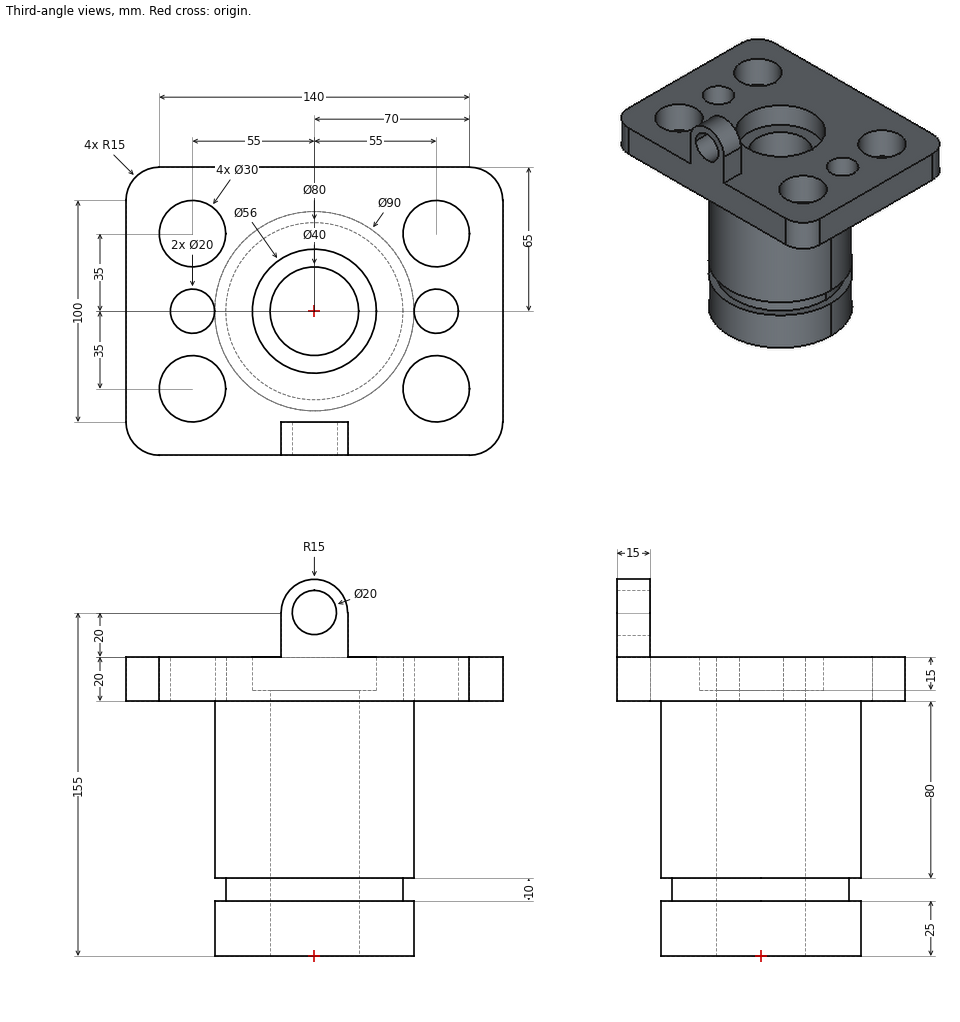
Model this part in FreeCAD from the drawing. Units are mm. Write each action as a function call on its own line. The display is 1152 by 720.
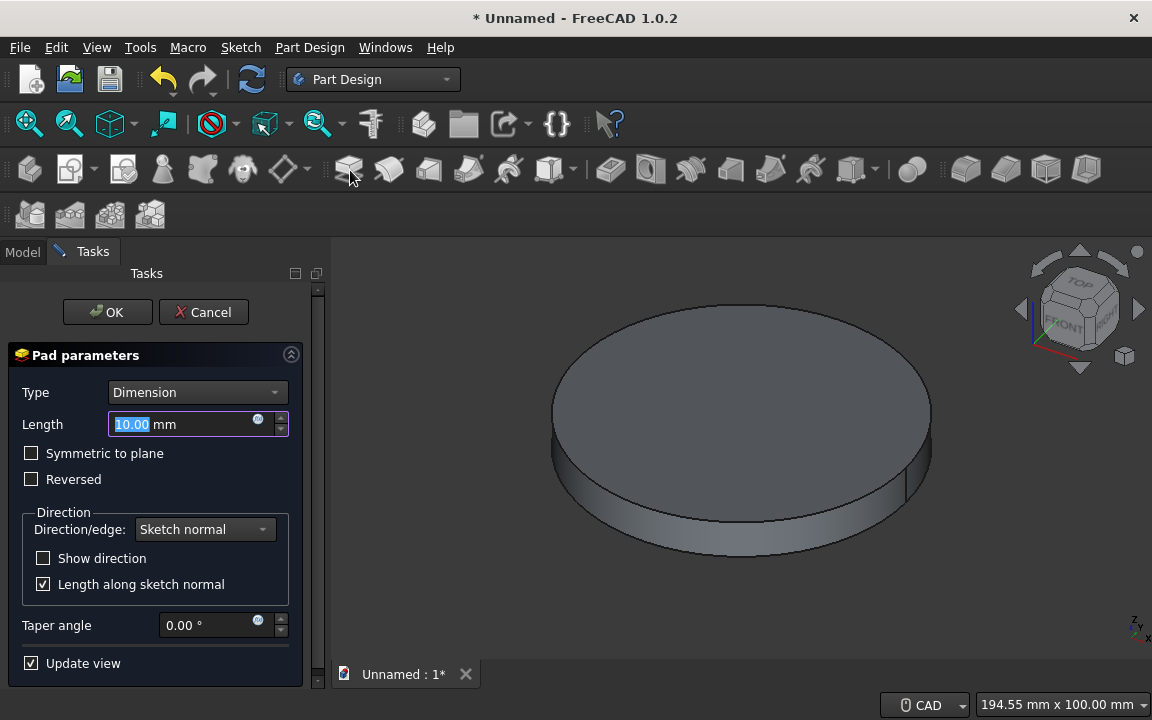
text(25)
key(Tab)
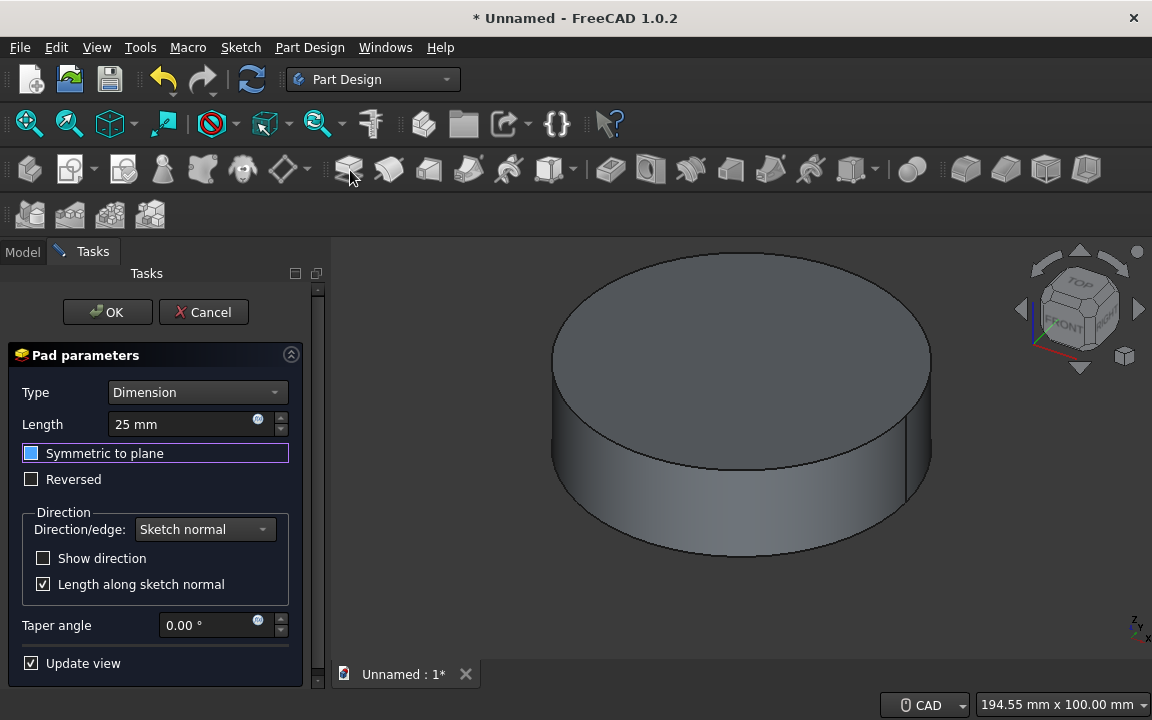
click(108, 312)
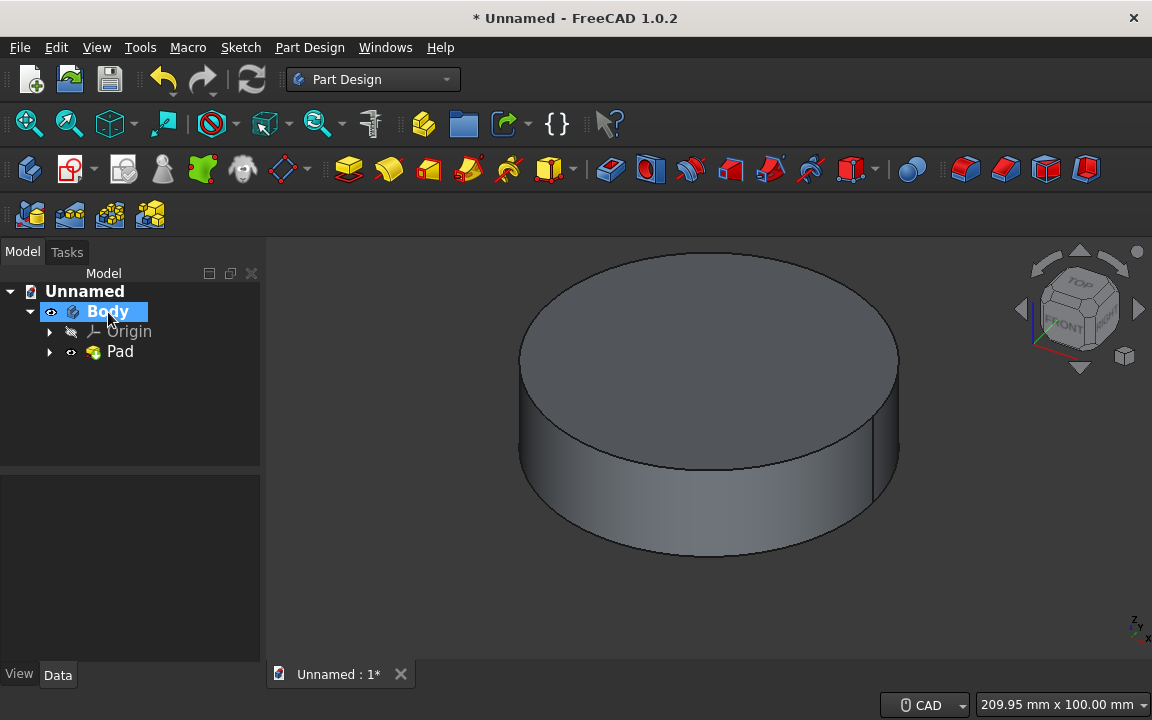
click(30, 124)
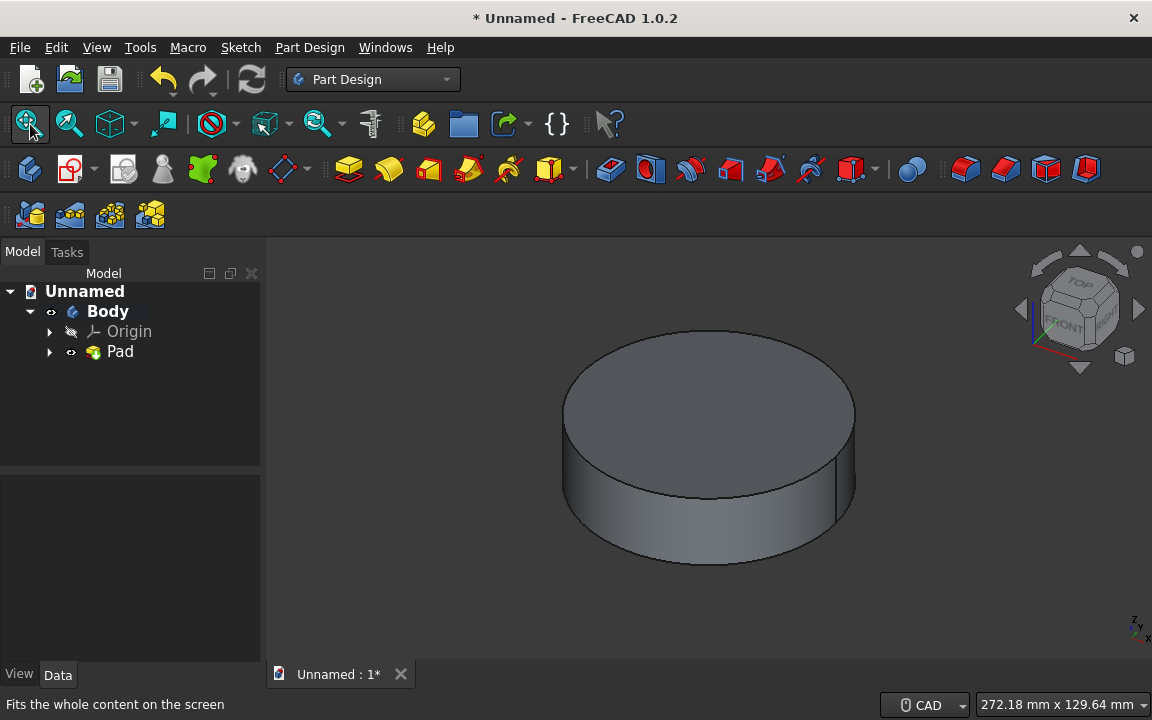
click(709, 414)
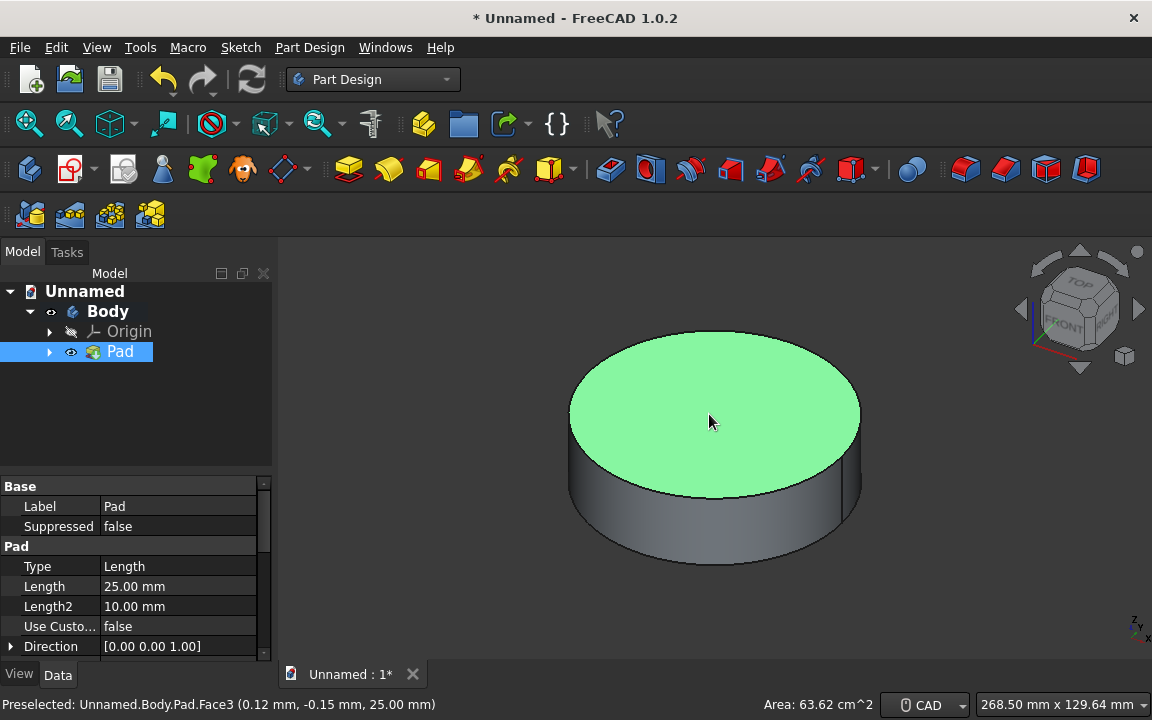
click(70, 170)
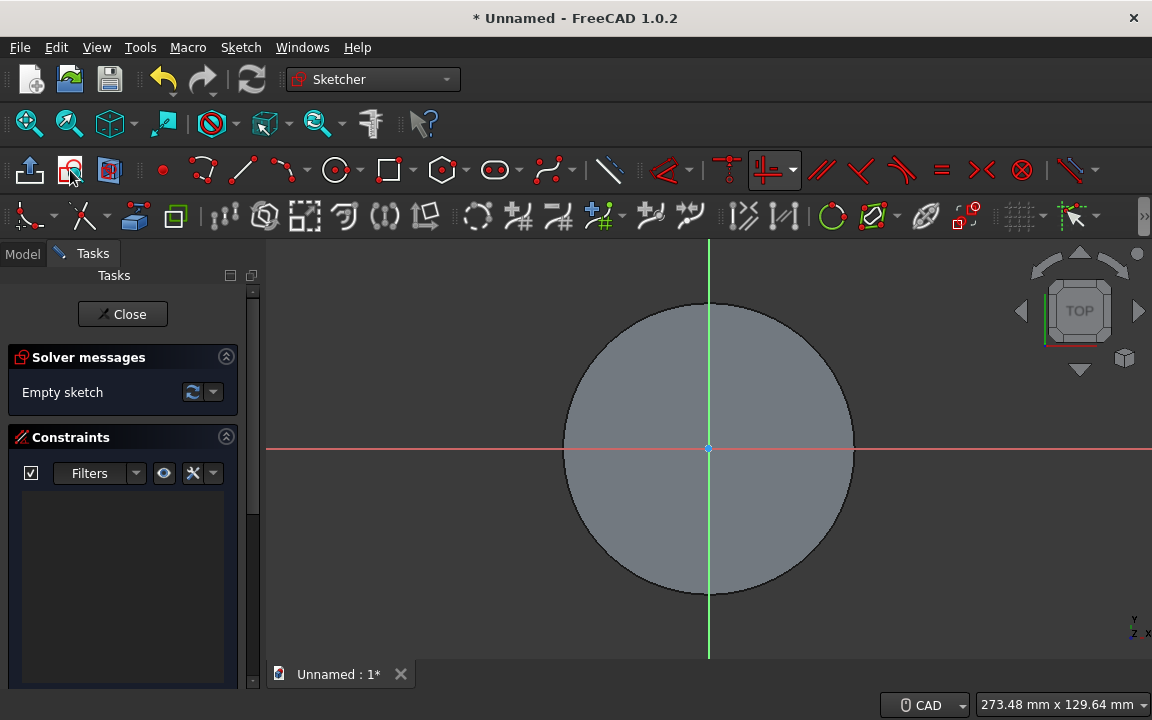
click(336, 170)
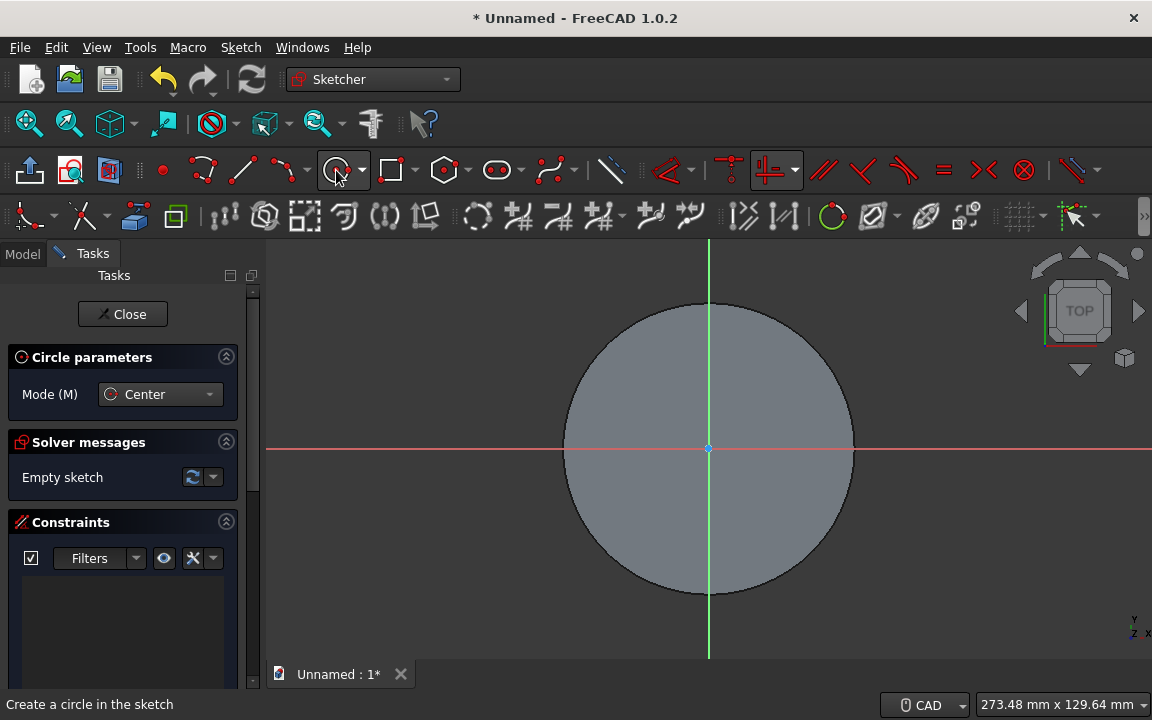
click(709, 449)
click(801, 357)
key(Escape)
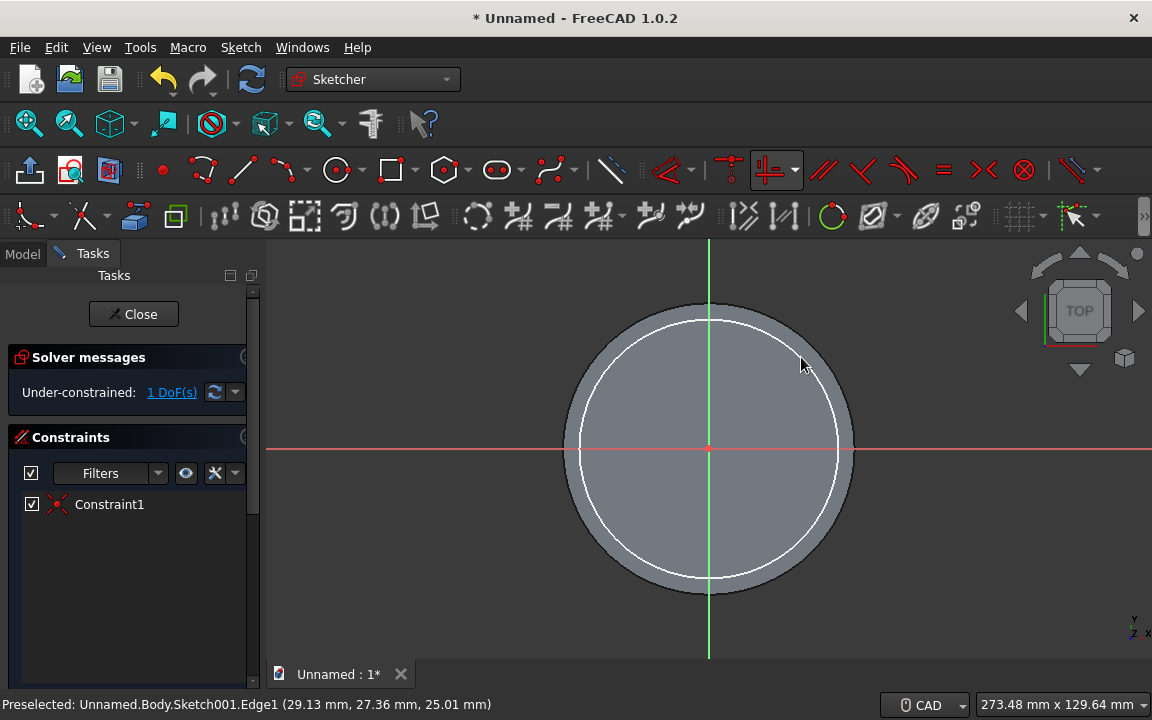
click(666, 170)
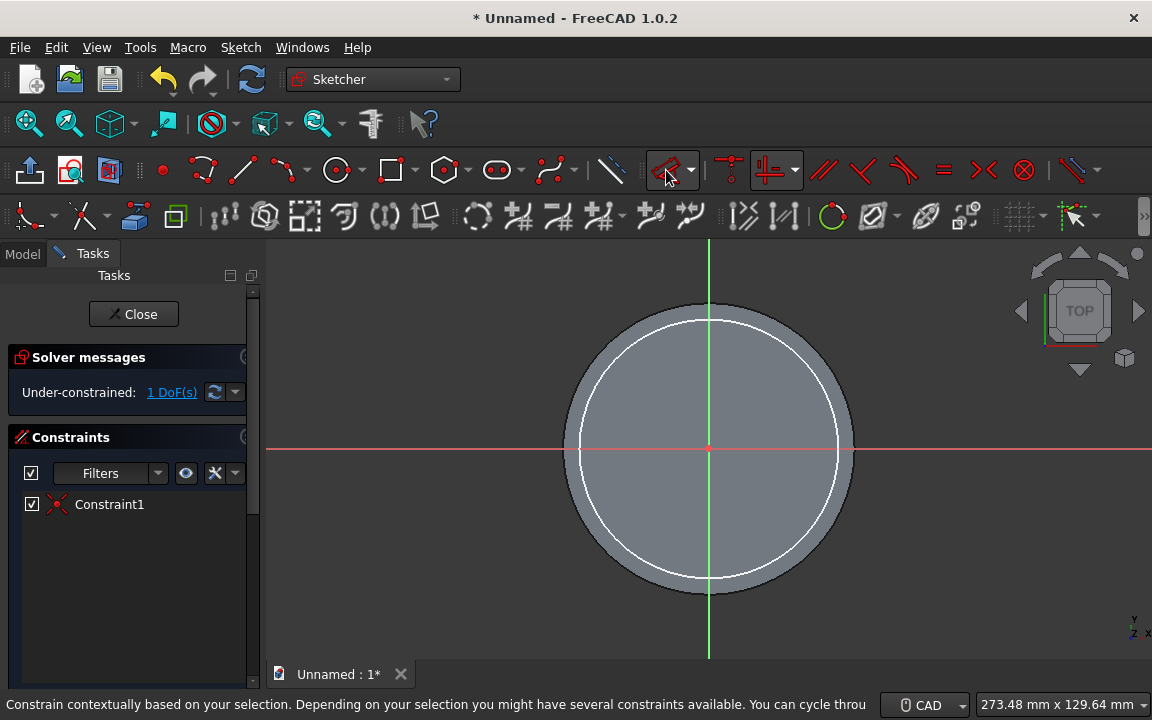
click(800, 357)
click(823, 334)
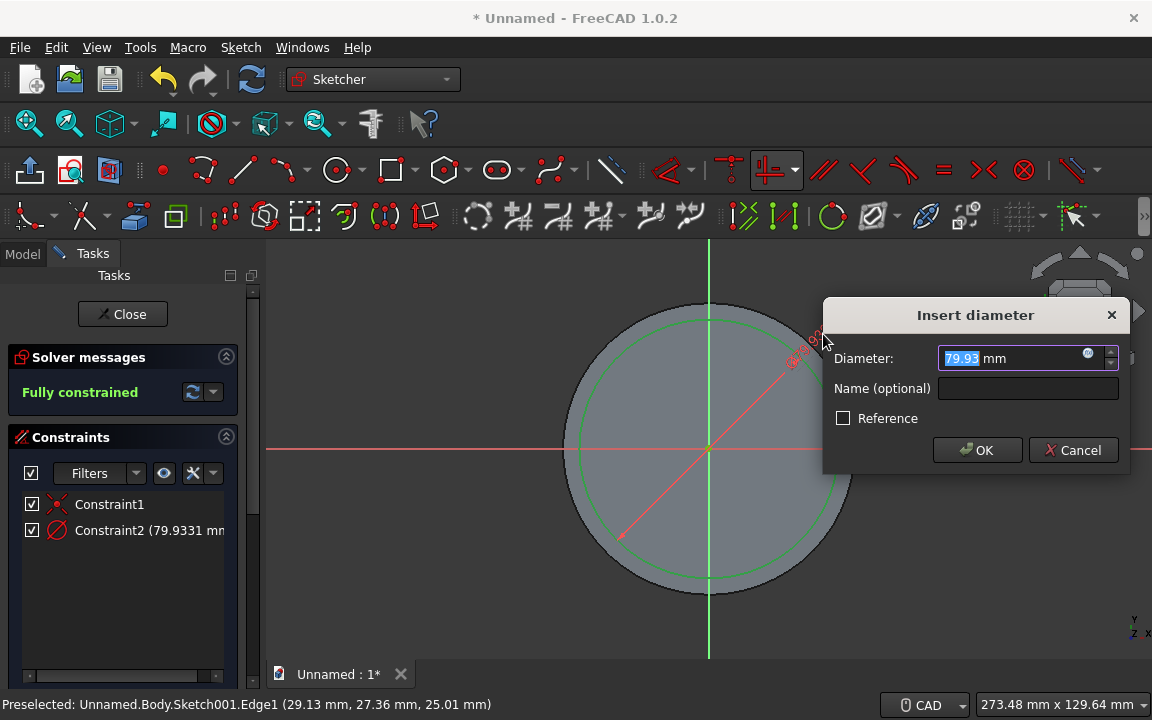
text(80)
key(Return)
key(Escape)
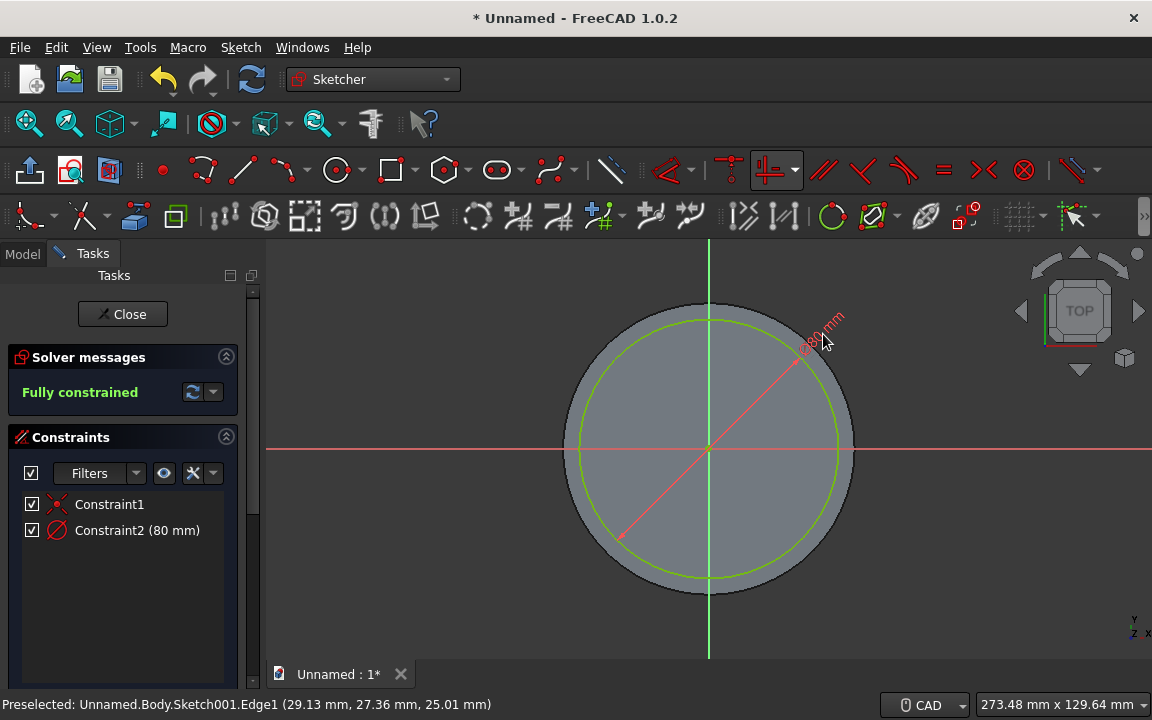
click(123, 314)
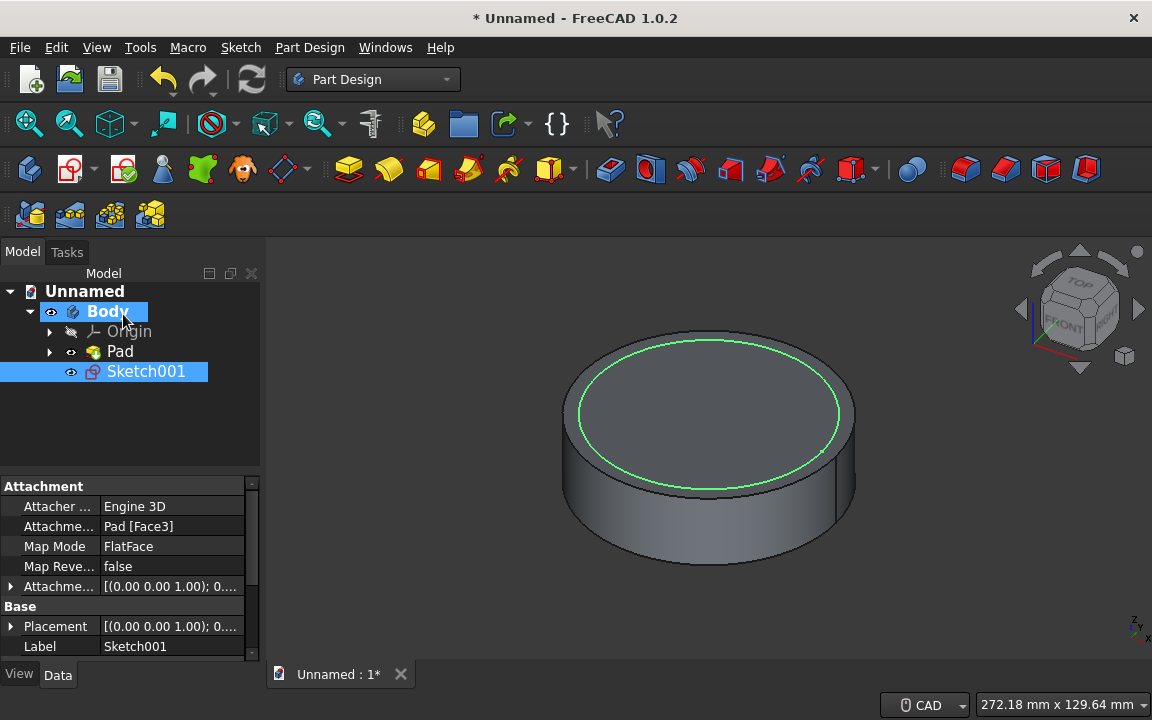
click(350, 170)